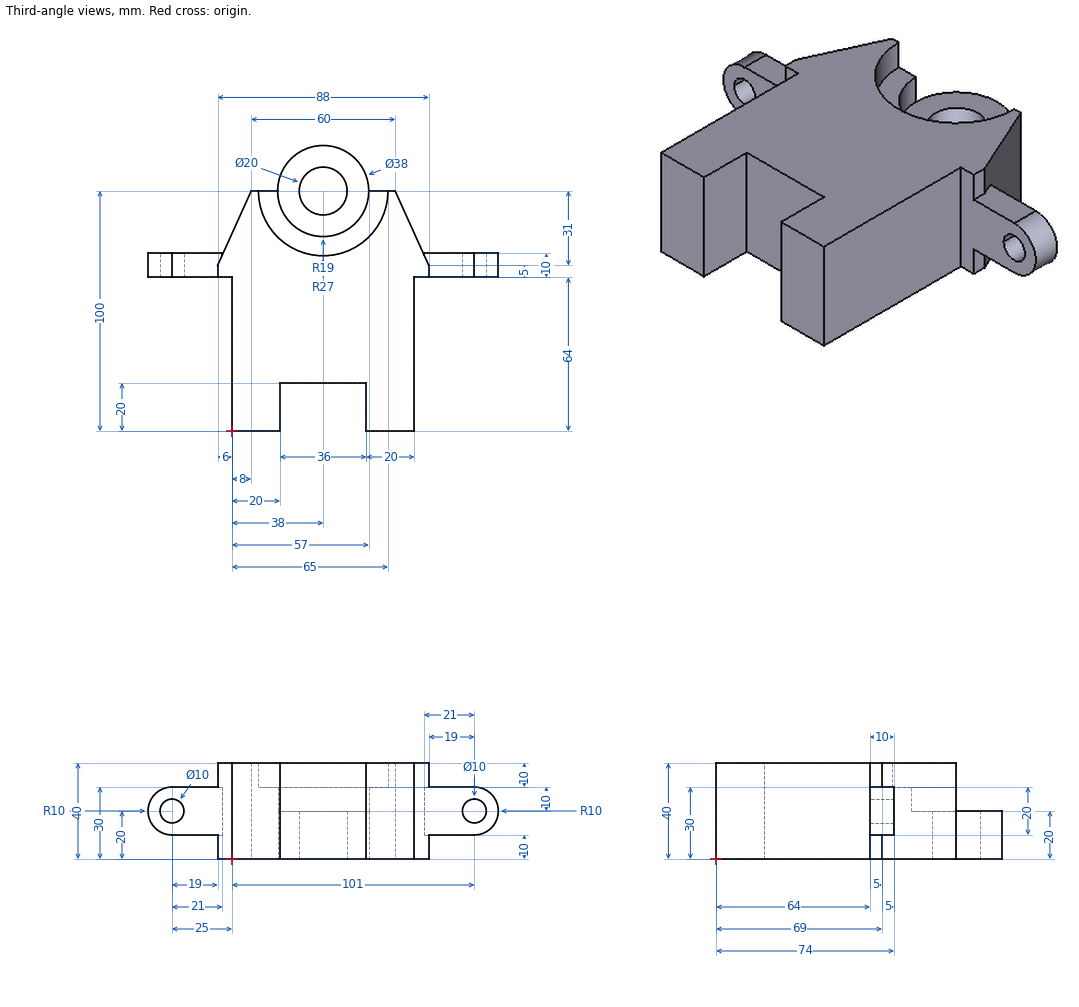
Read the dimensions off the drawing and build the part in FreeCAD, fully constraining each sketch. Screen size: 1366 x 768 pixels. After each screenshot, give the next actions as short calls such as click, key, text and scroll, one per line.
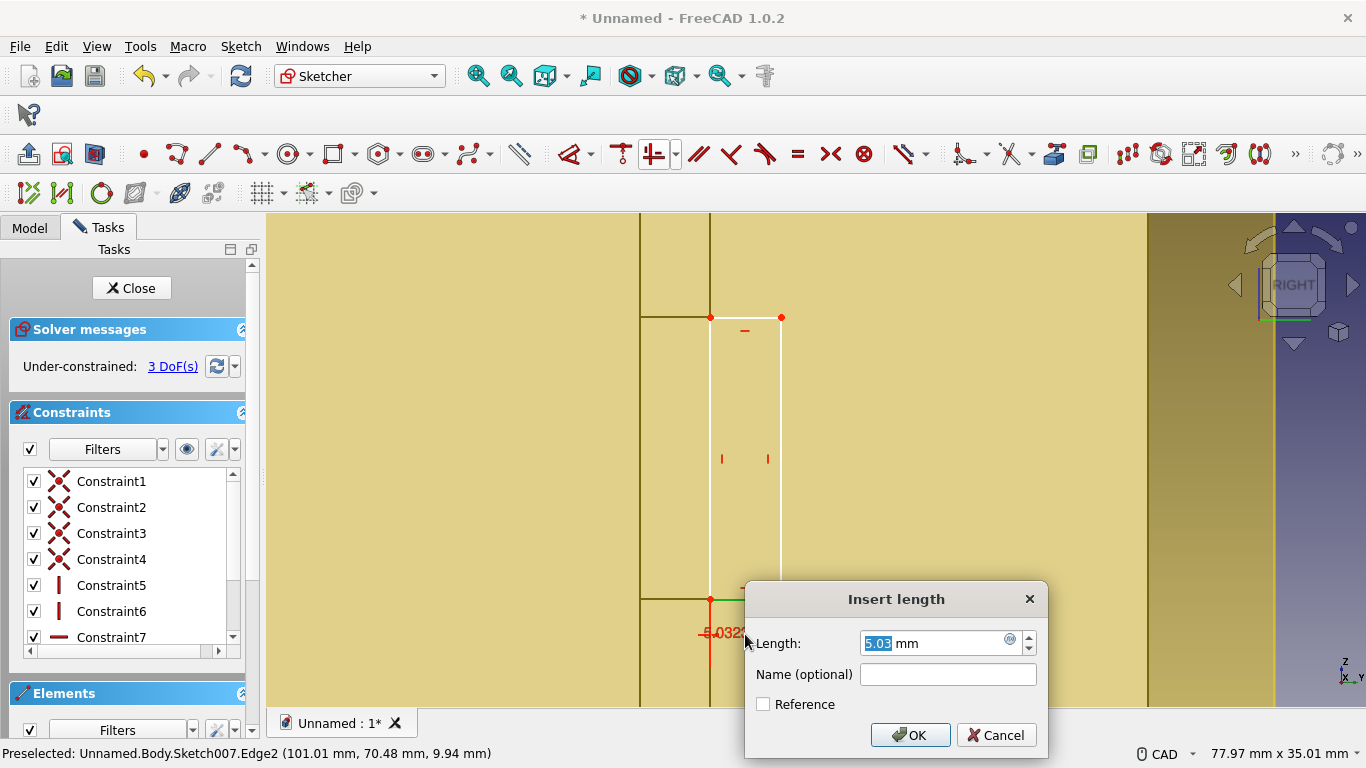
text(5)
key(Return)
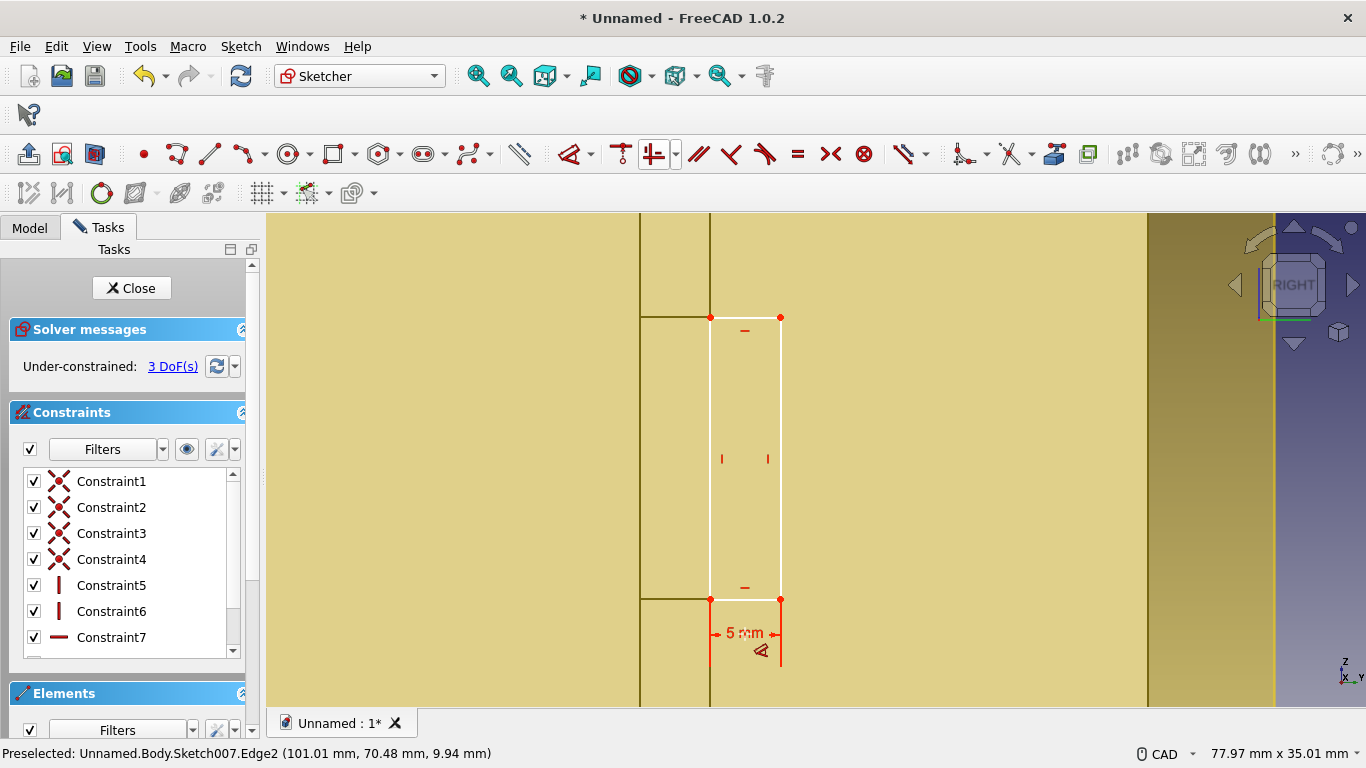
click(710, 403)
click(676, 459)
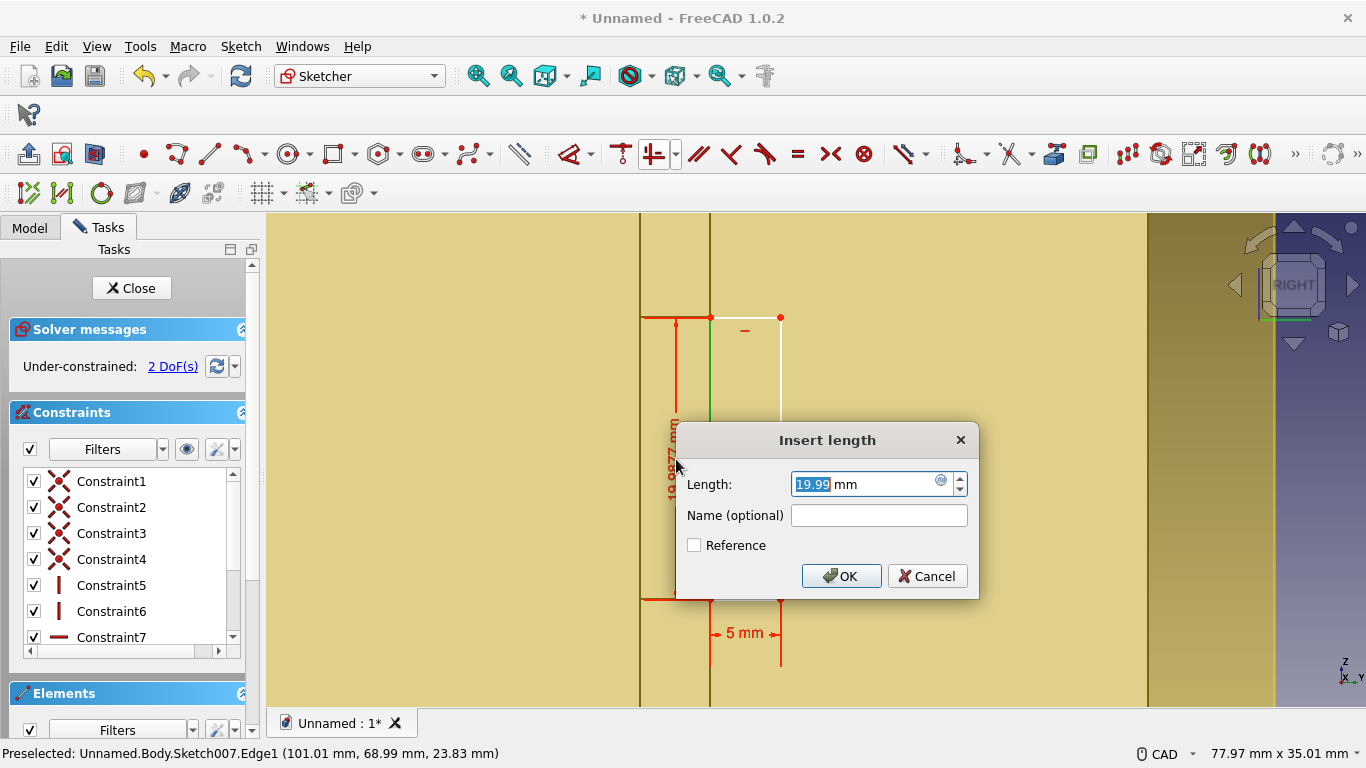
text(20)
key(Return)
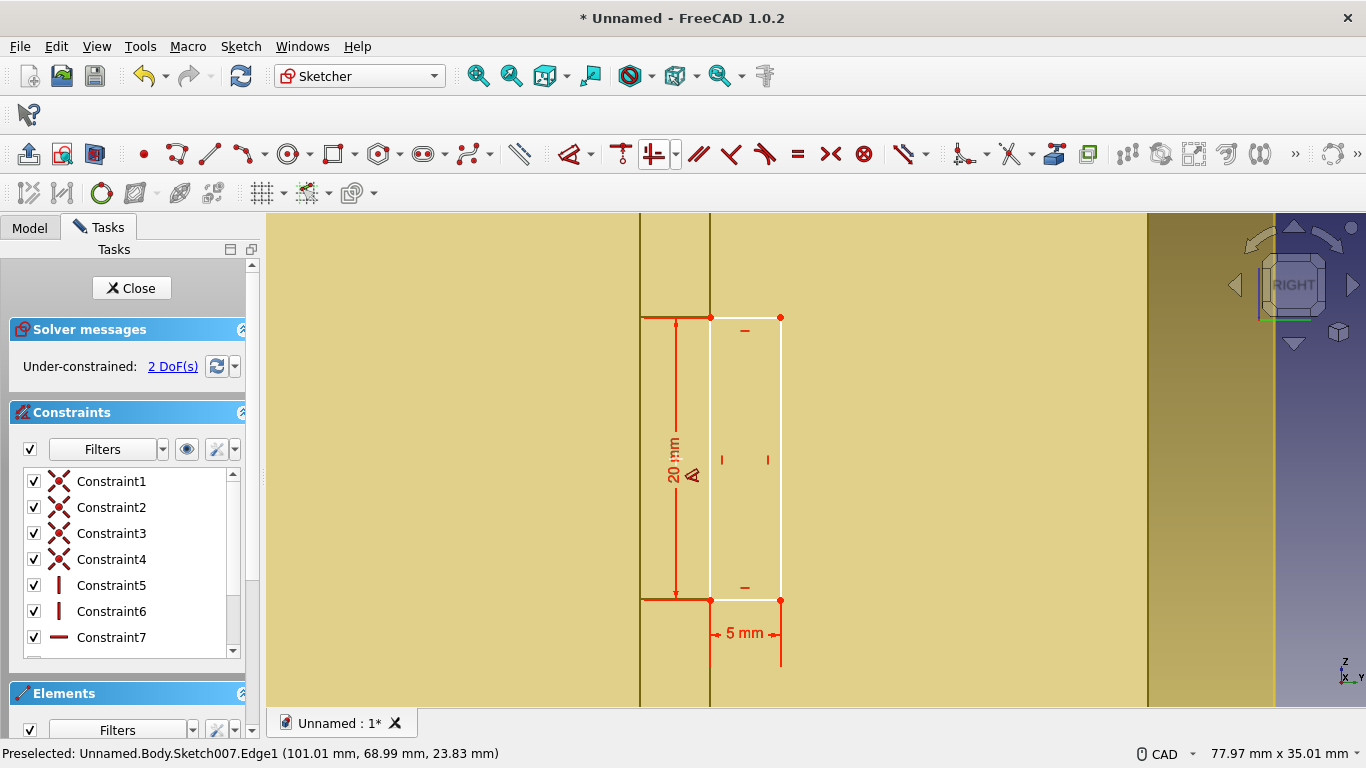
click(710, 318)
click(502, 284)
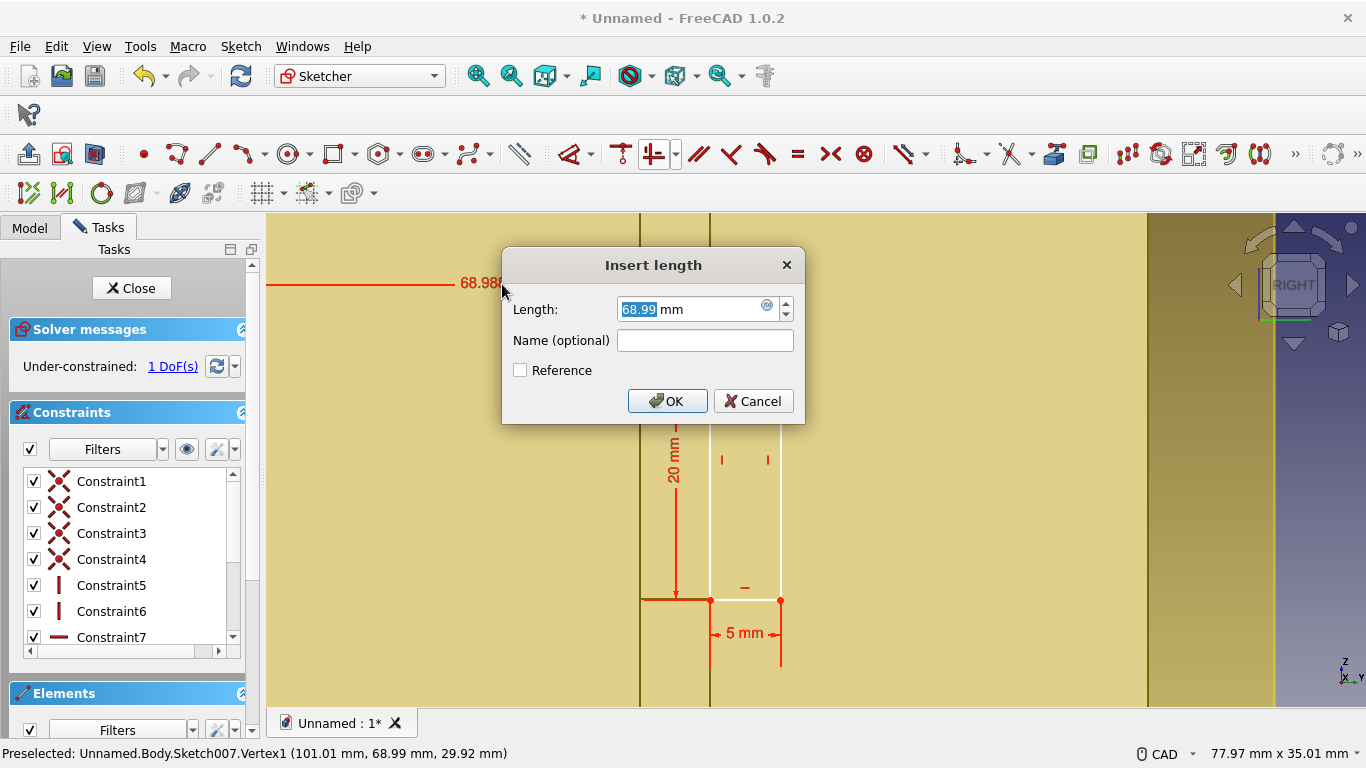
text(69)
key(Return)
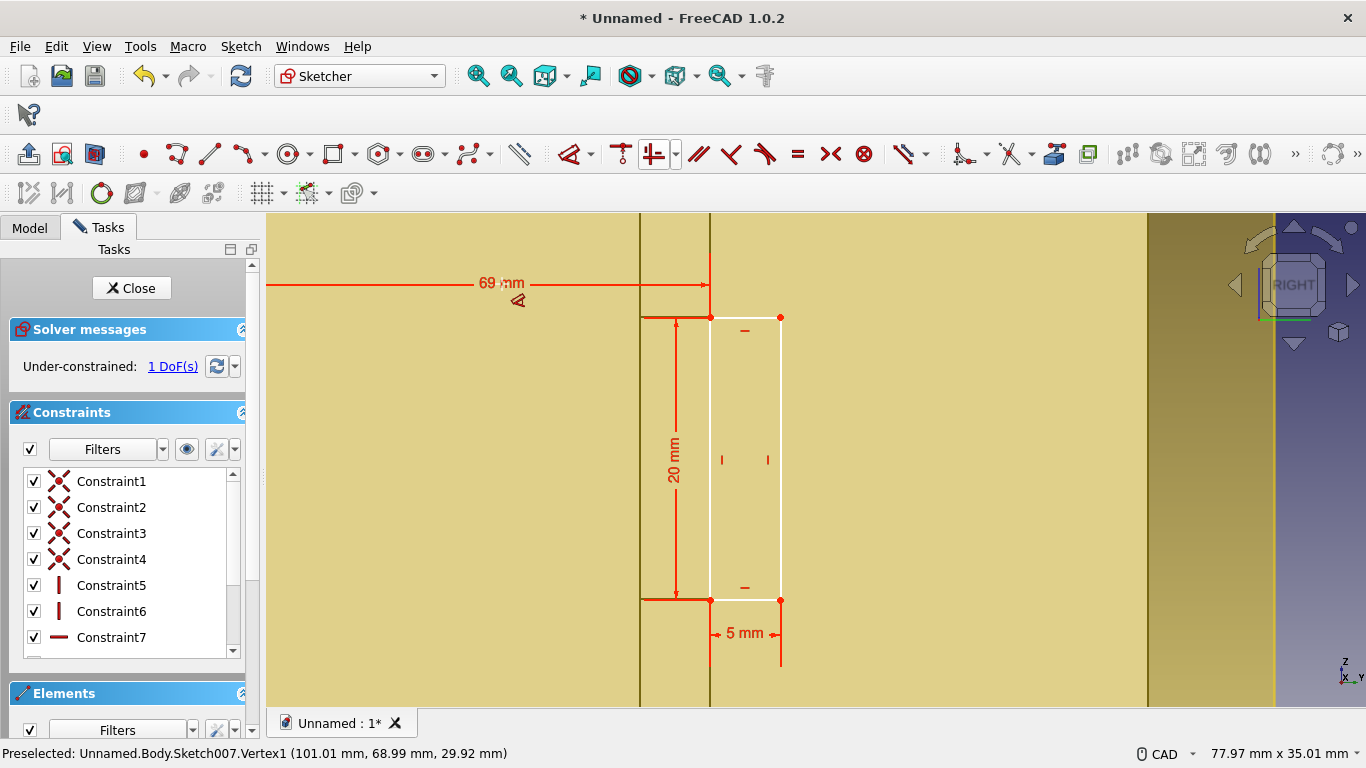
click(710, 318)
click(744, 498)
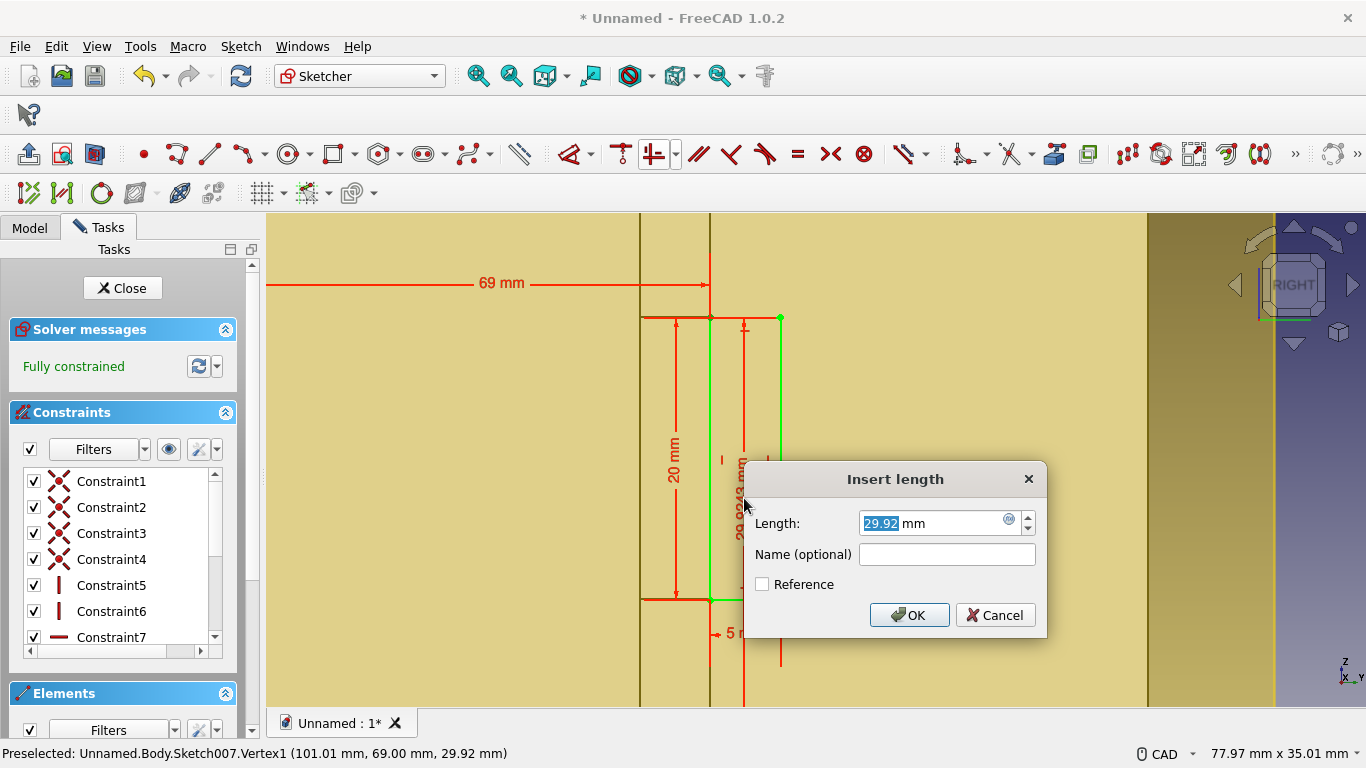
text(30)
key(Return)
key(Escape)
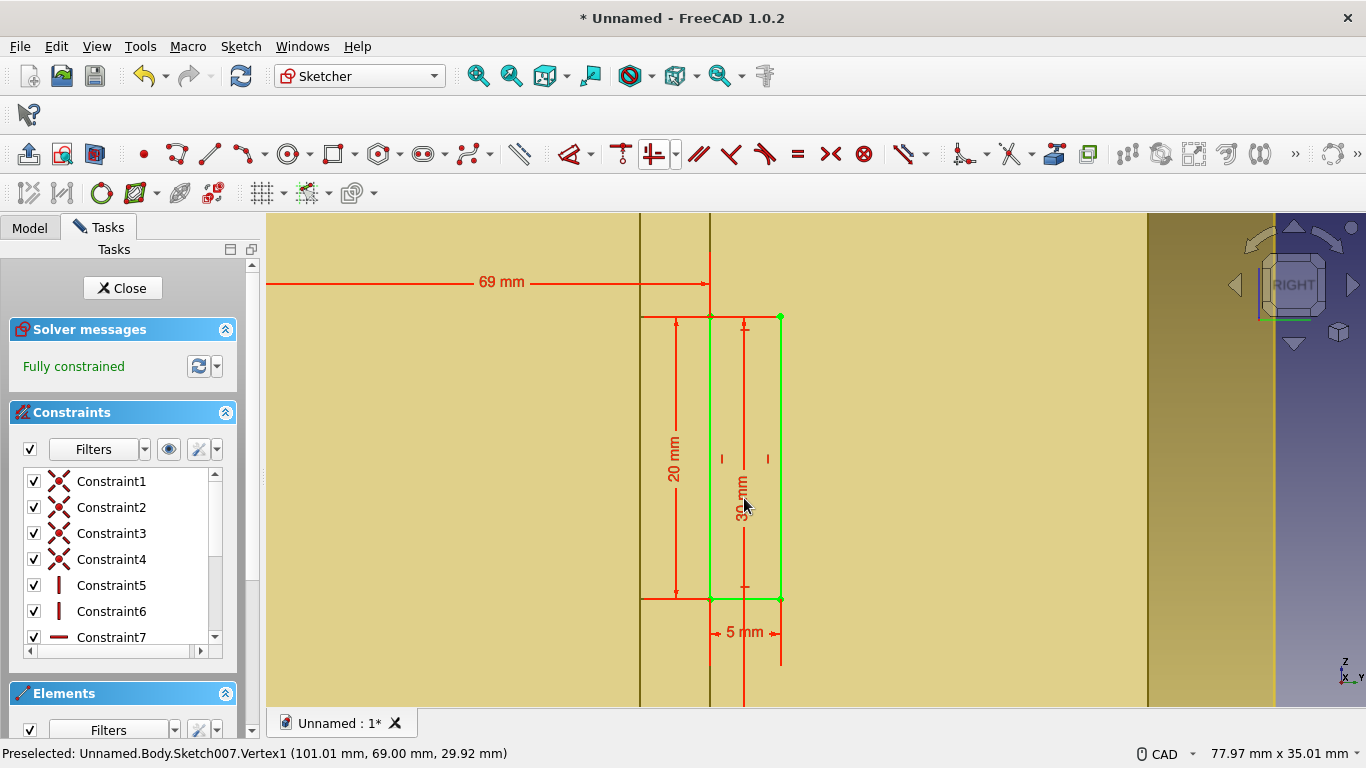
click(123, 288)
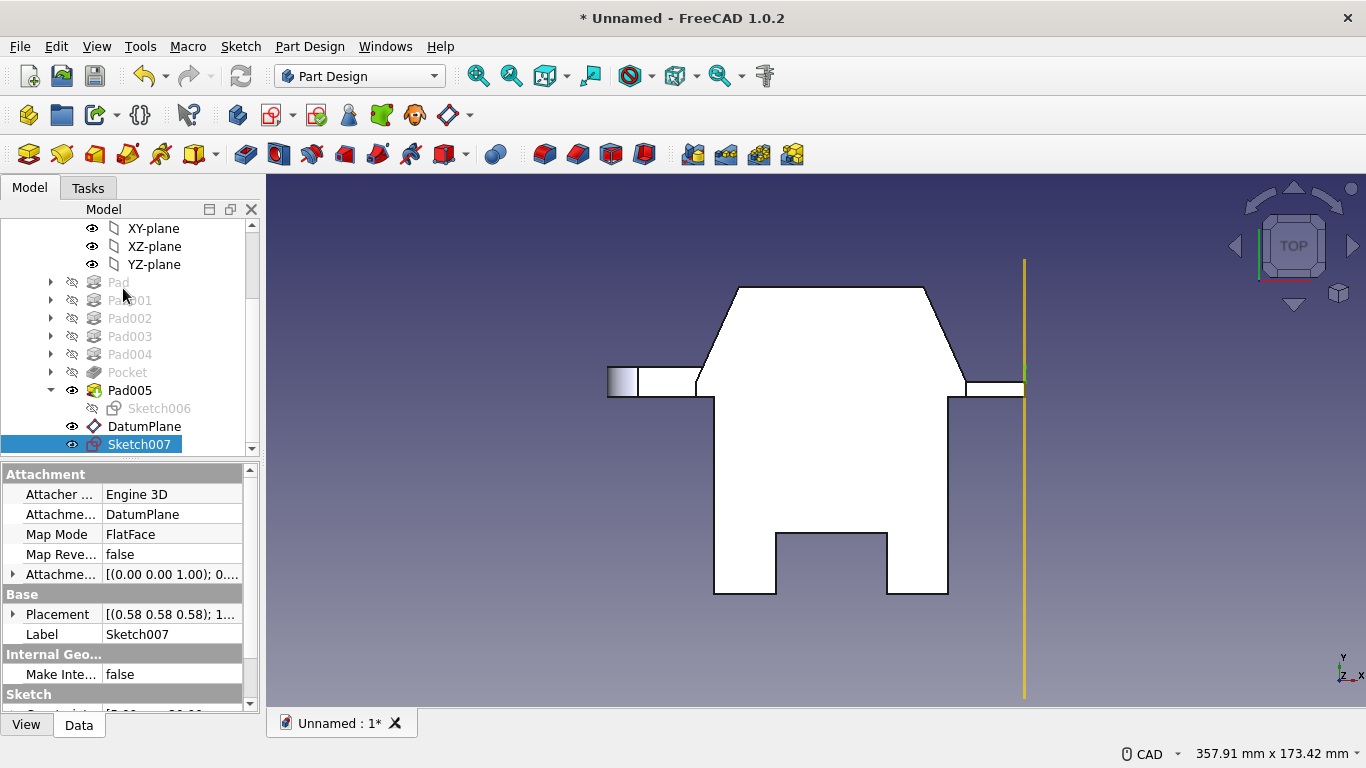
click(29, 154)